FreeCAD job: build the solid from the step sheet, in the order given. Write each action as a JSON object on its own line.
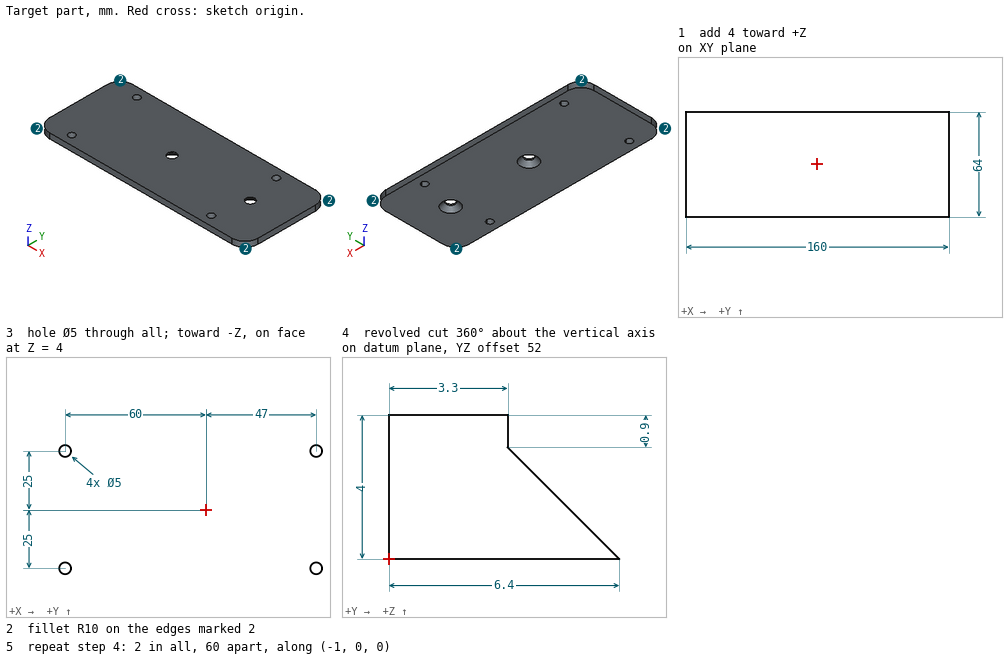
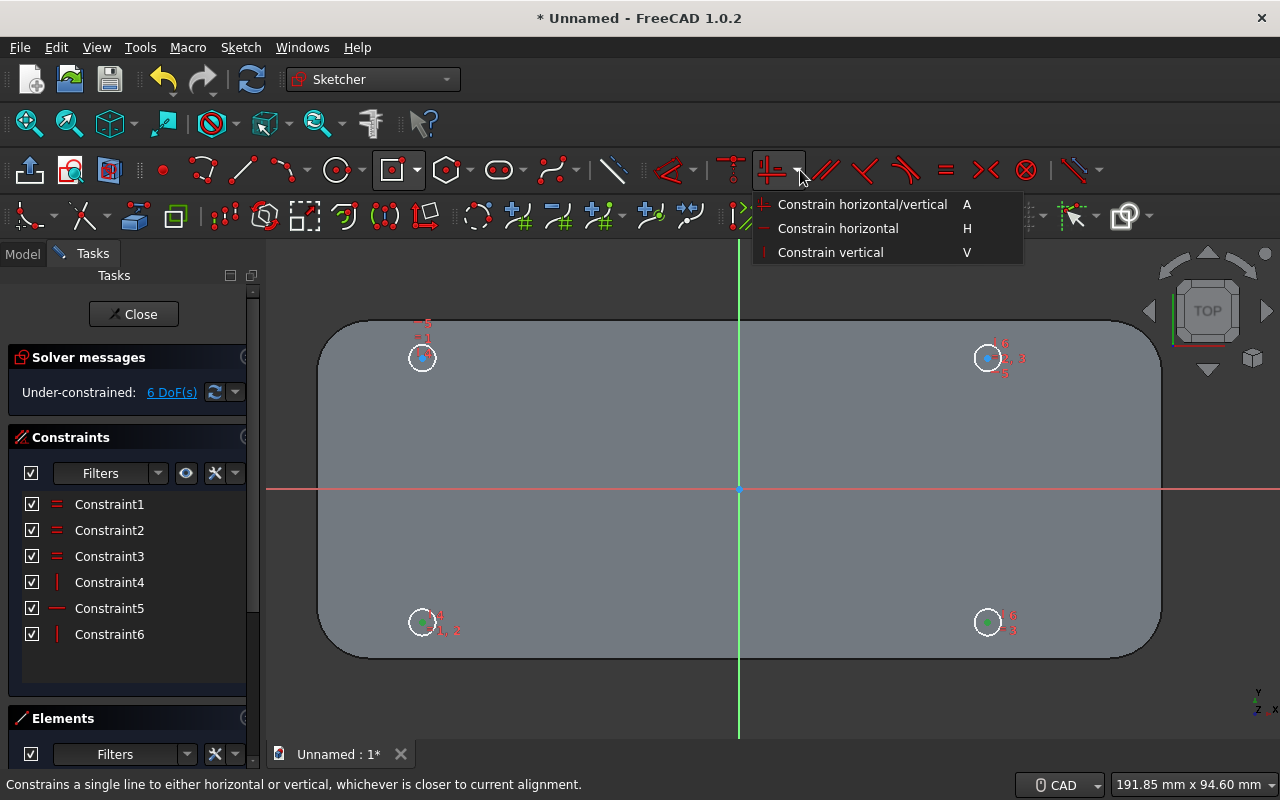
{"action": "left_click", "coordinate": [888, 228]}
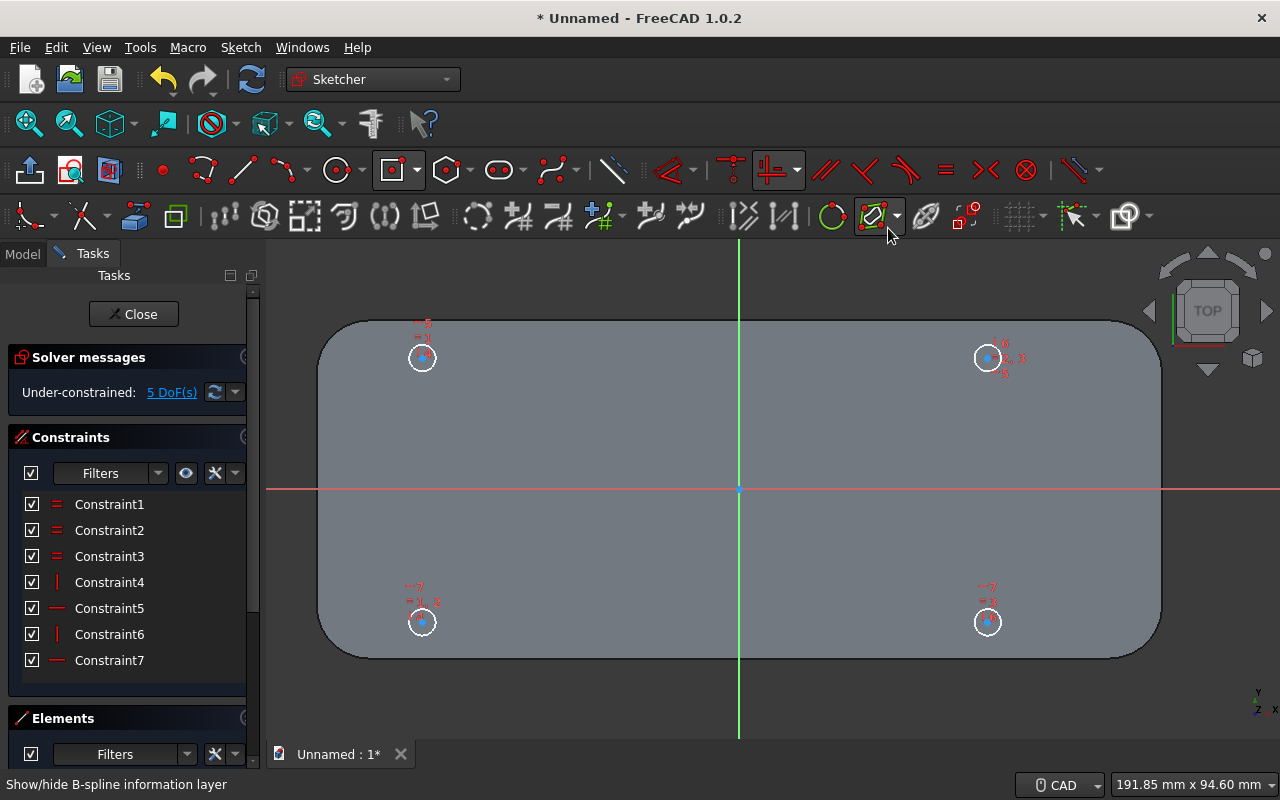
{"action": "left_click", "coordinate": [668, 170]}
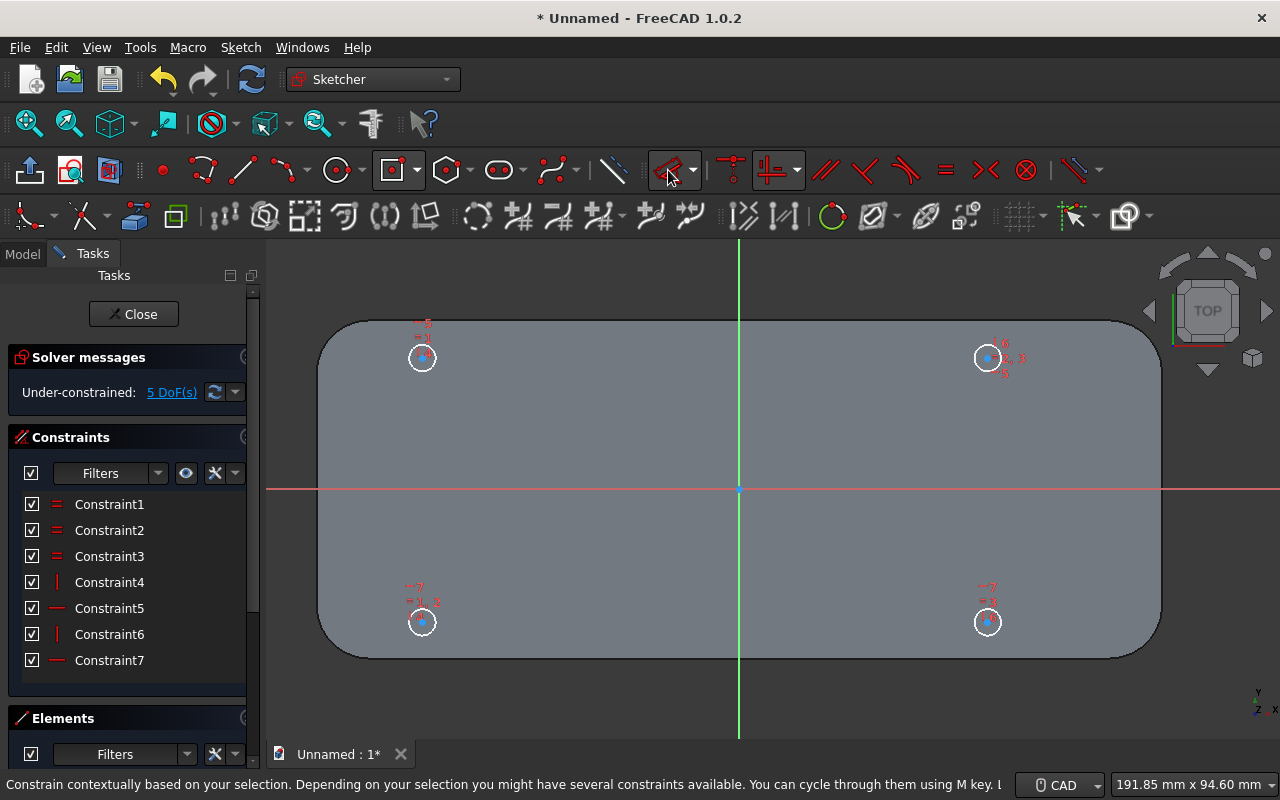
{"action": "scroll", "coordinate": [432, 349], "scroll_direction": "up", "scroll_amount": 3}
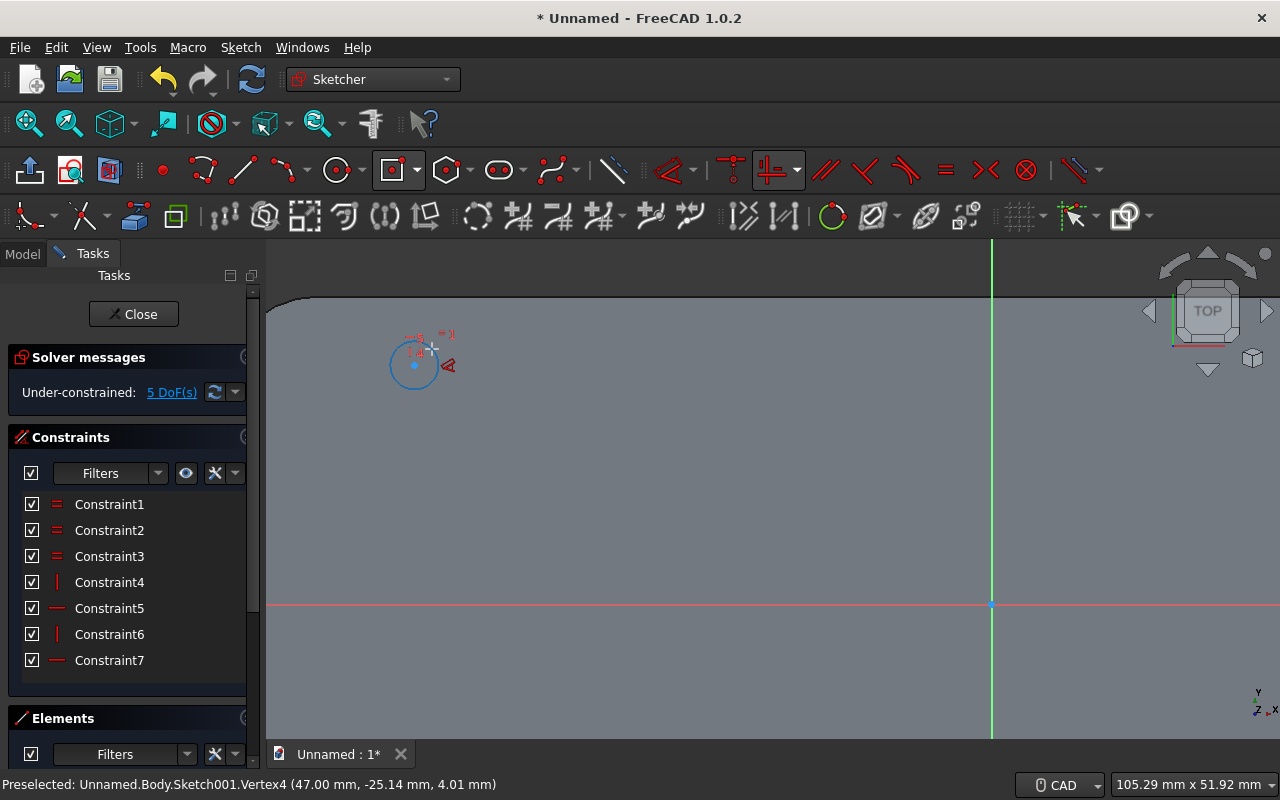
{"action": "left_click", "coordinate": [431, 348]}
{"action": "left_click", "coordinate": [453, 325]}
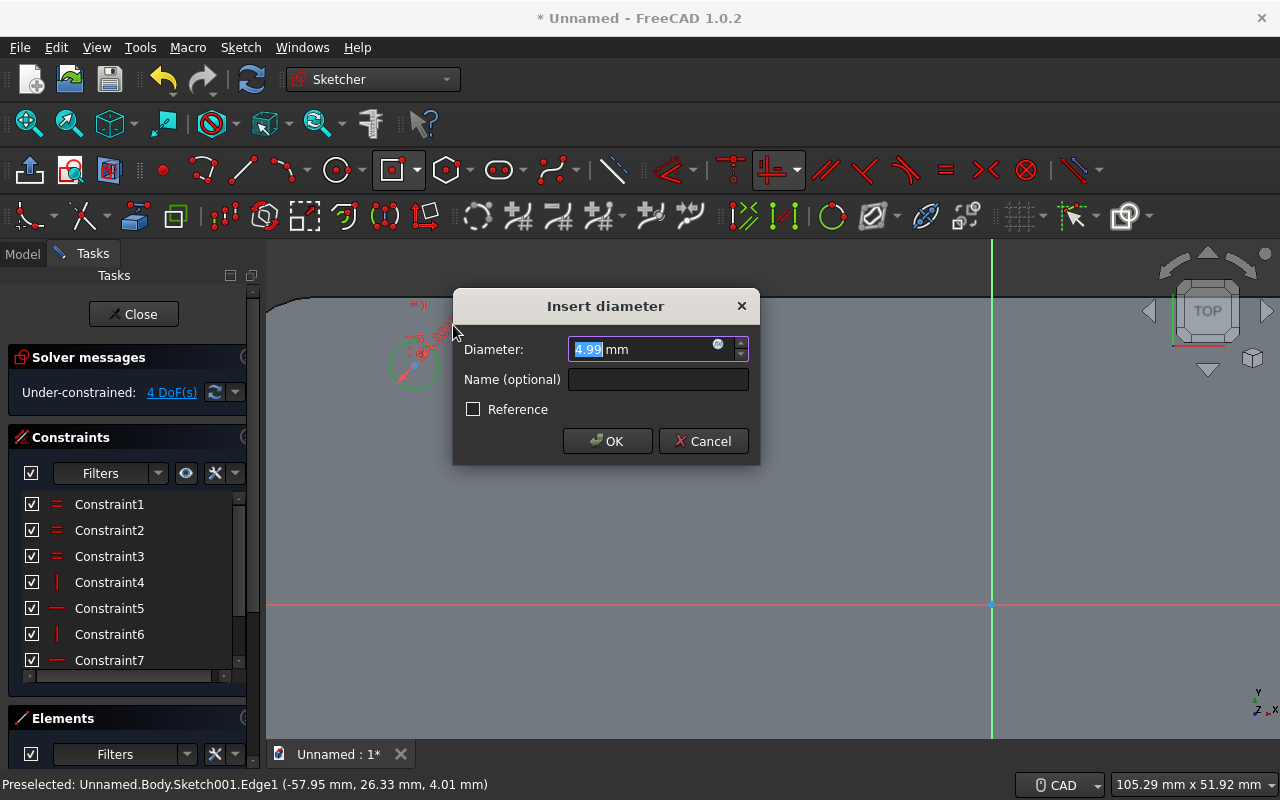
{"action": "type", "text": "5"}
{"action": "key", "text": "Return"}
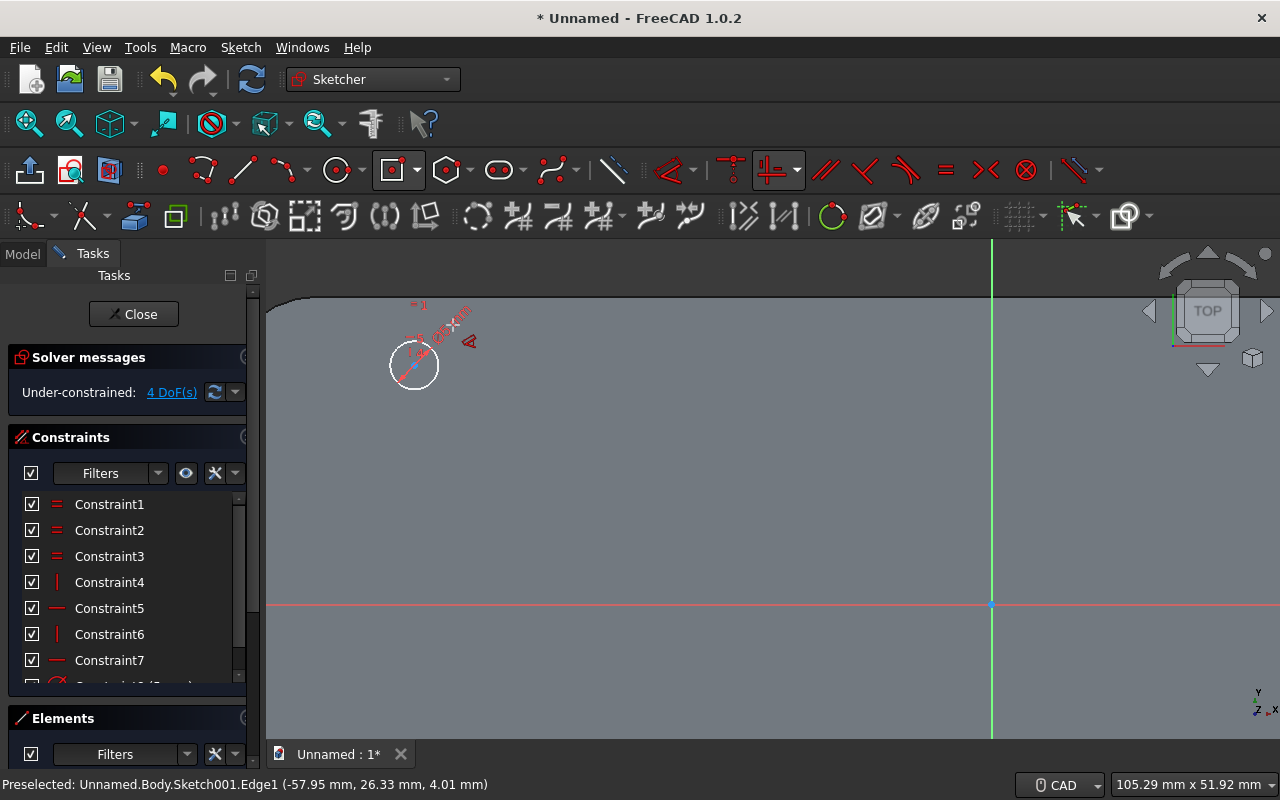
{"action": "left_click", "coordinate": [414, 365]}
{"action": "left_click", "coordinate": [703, 331]}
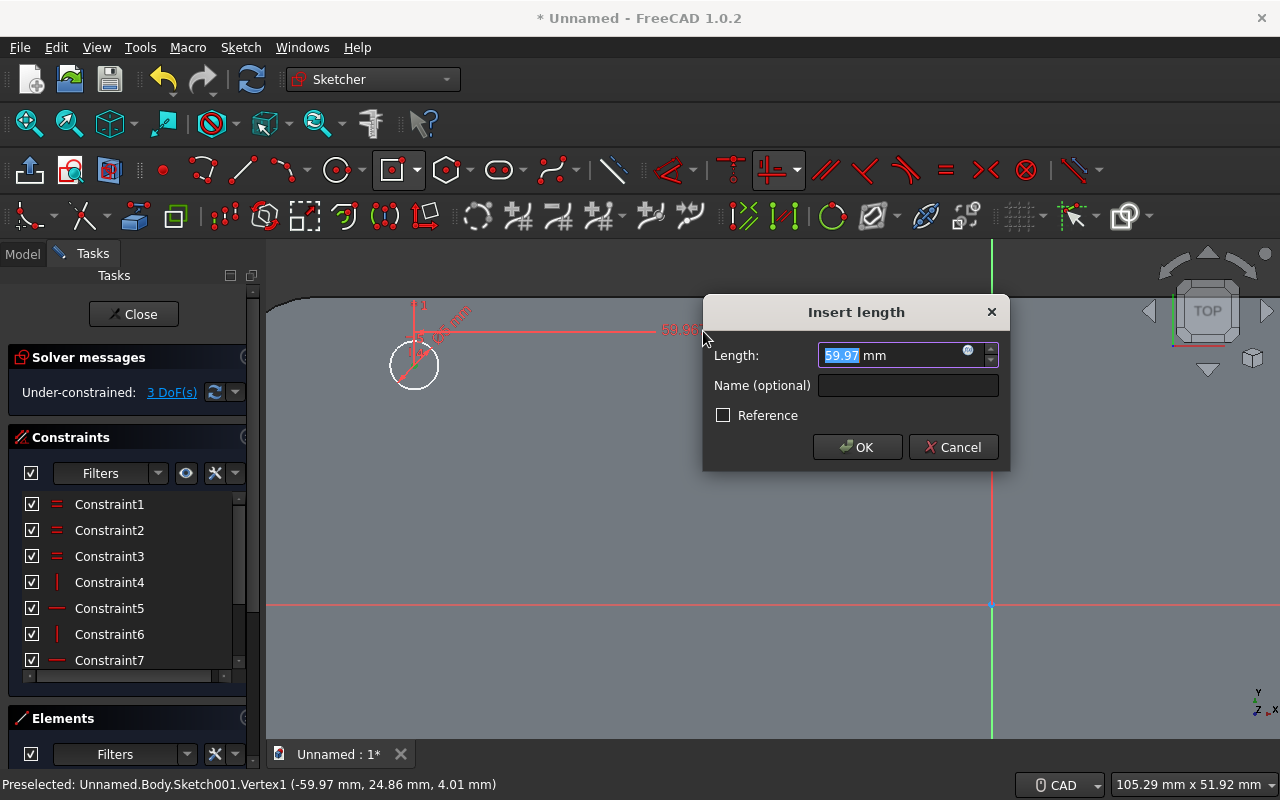
{"action": "type", "text": "60"}
{"action": "key", "text": "Return"}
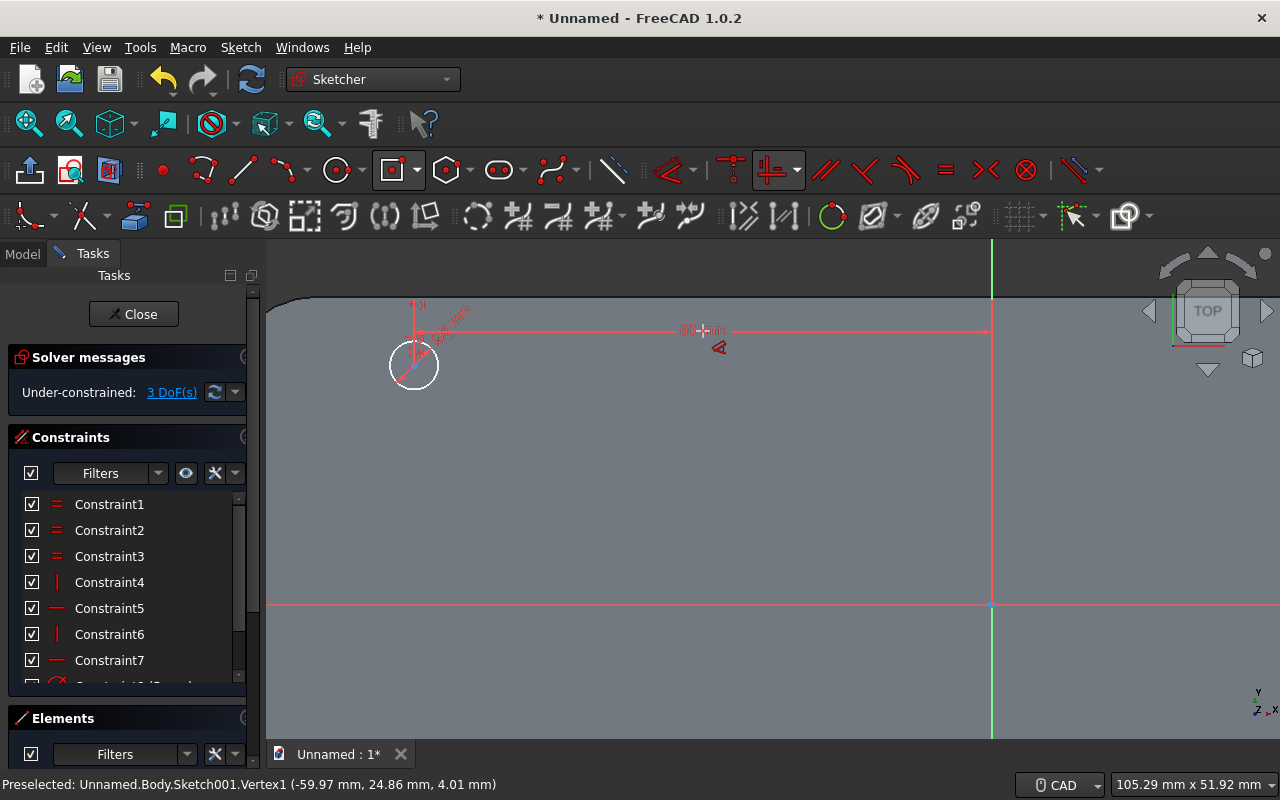
{"action": "left_click", "coordinate": [414, 365]}
{"action": "left_click", "coordinate": [380, 485]}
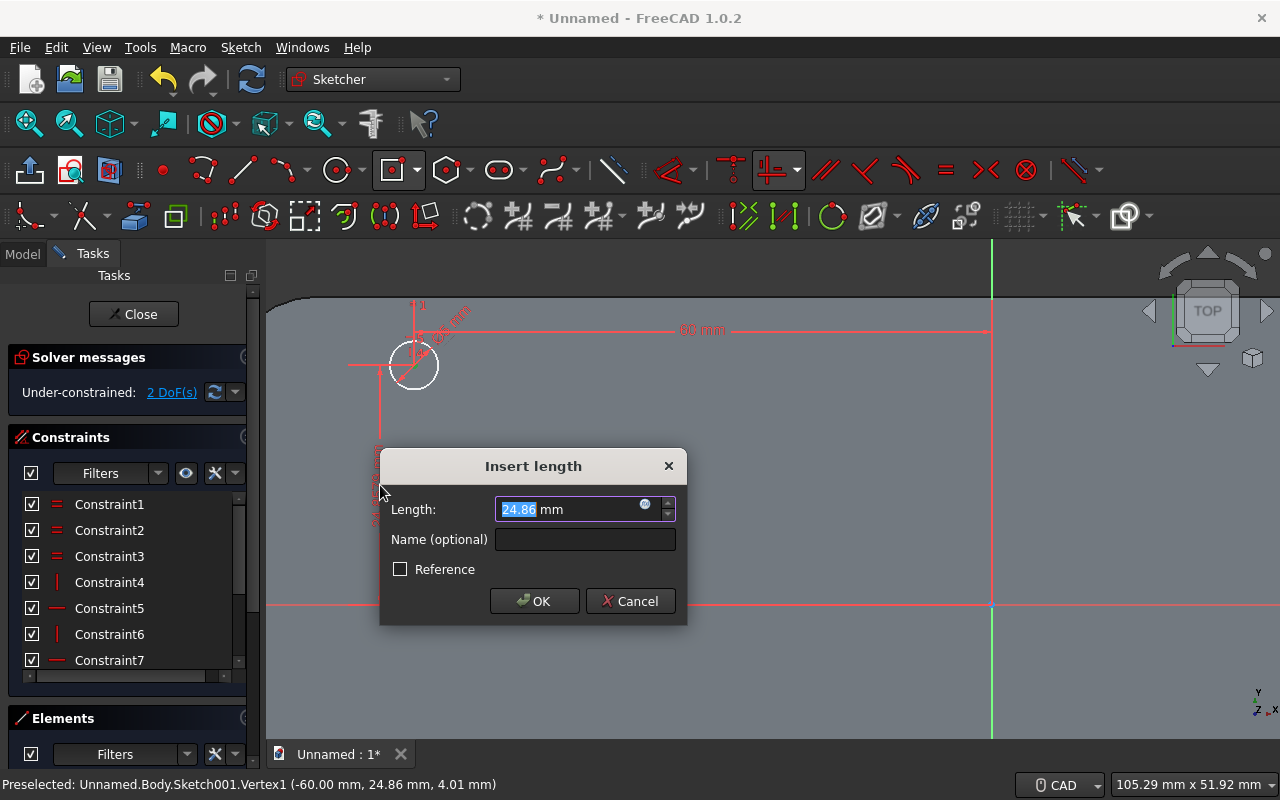
{"action": "type", "text": "25"}
{"action": "key", "text": "Return"}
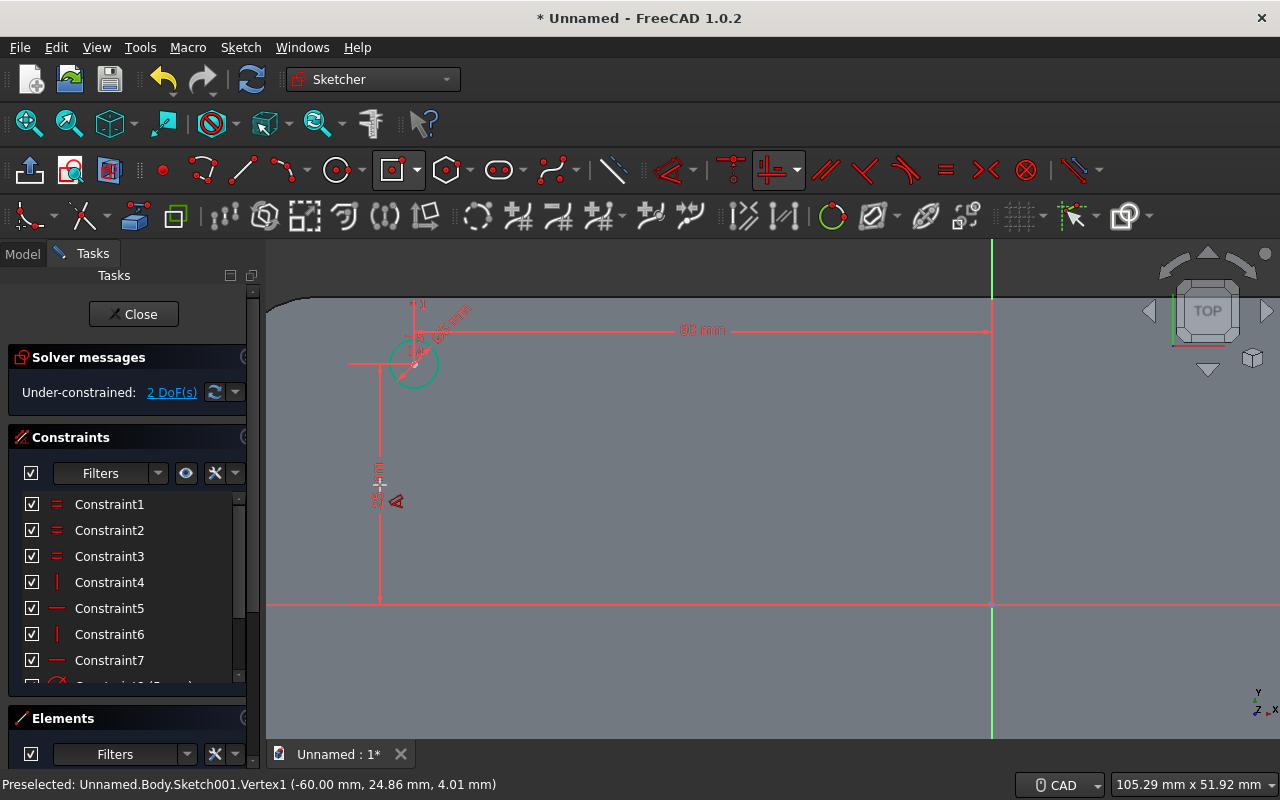
{"action": "scroll", "coordinate": [431, 348], "scroll_direction": "down", "scroll_amount": 3}